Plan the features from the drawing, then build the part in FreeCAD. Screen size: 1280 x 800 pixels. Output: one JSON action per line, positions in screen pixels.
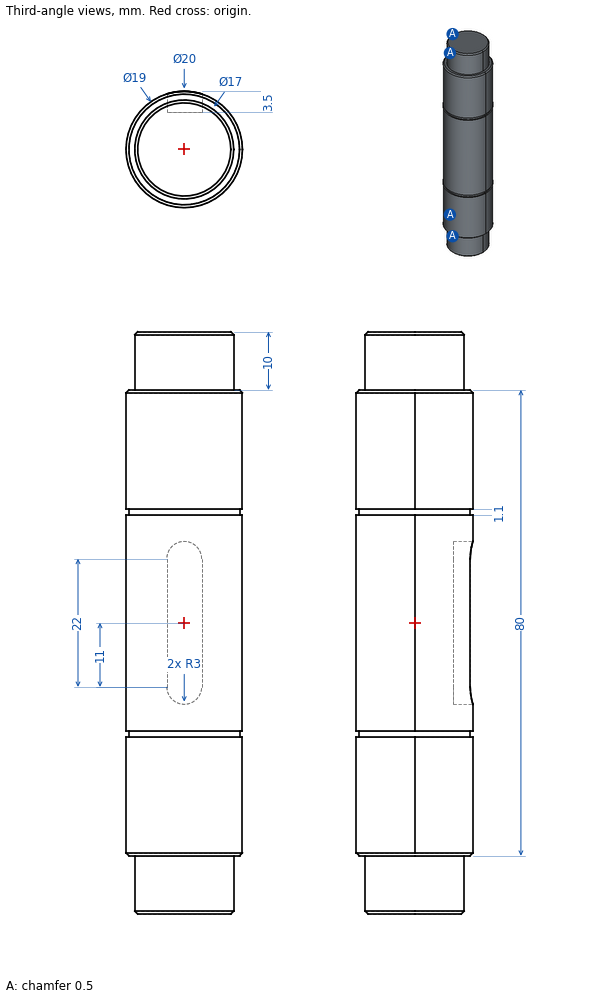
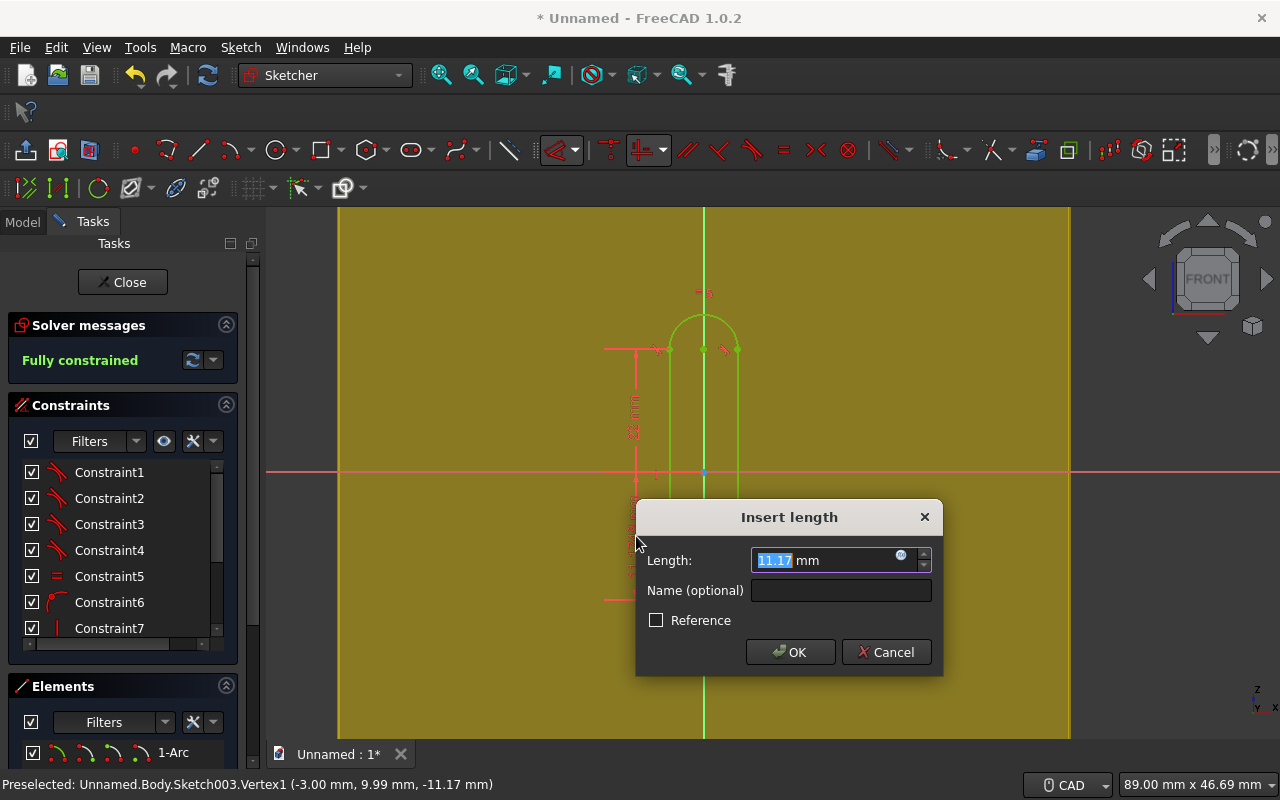
{"action": "type", "text": "11"}
{"action": "key", "text": "Return"}
{"action": "key", "text": "Escape"}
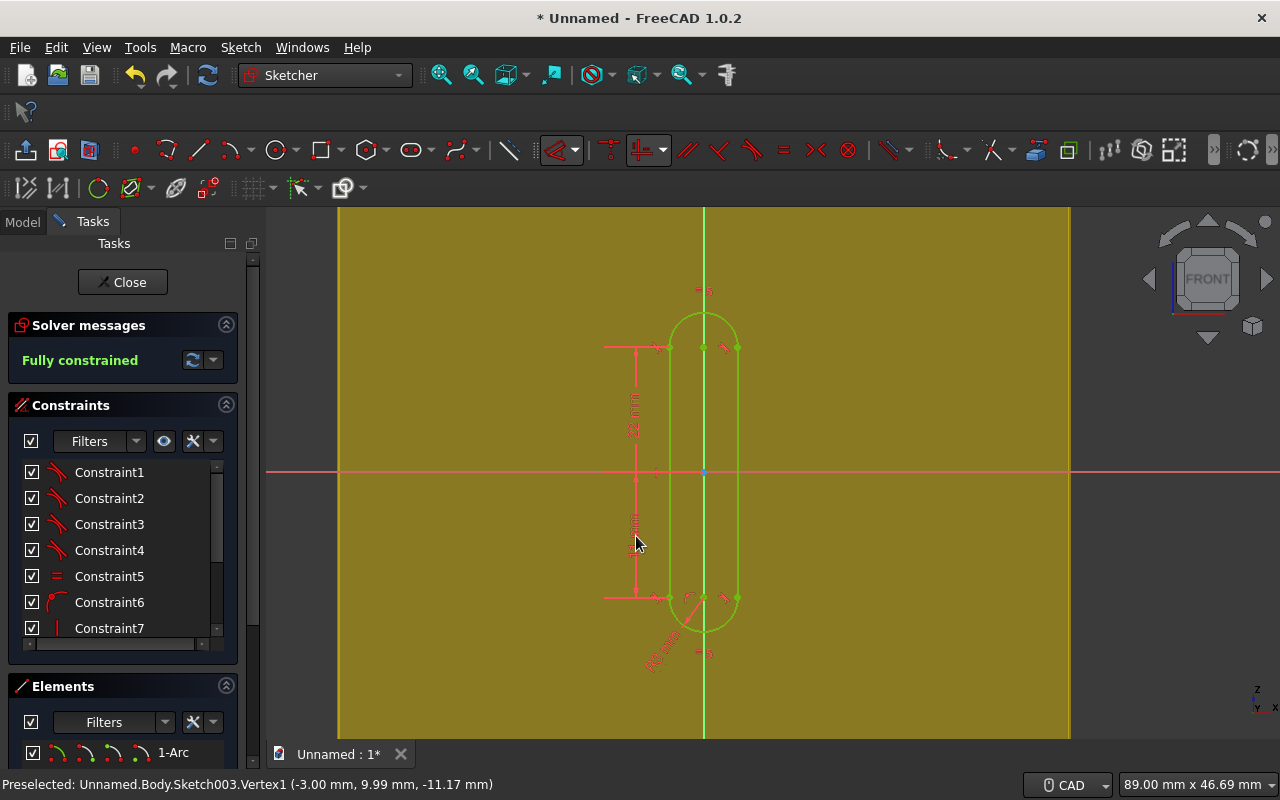
{"action": "left_click", "coordinate": [123, 282]}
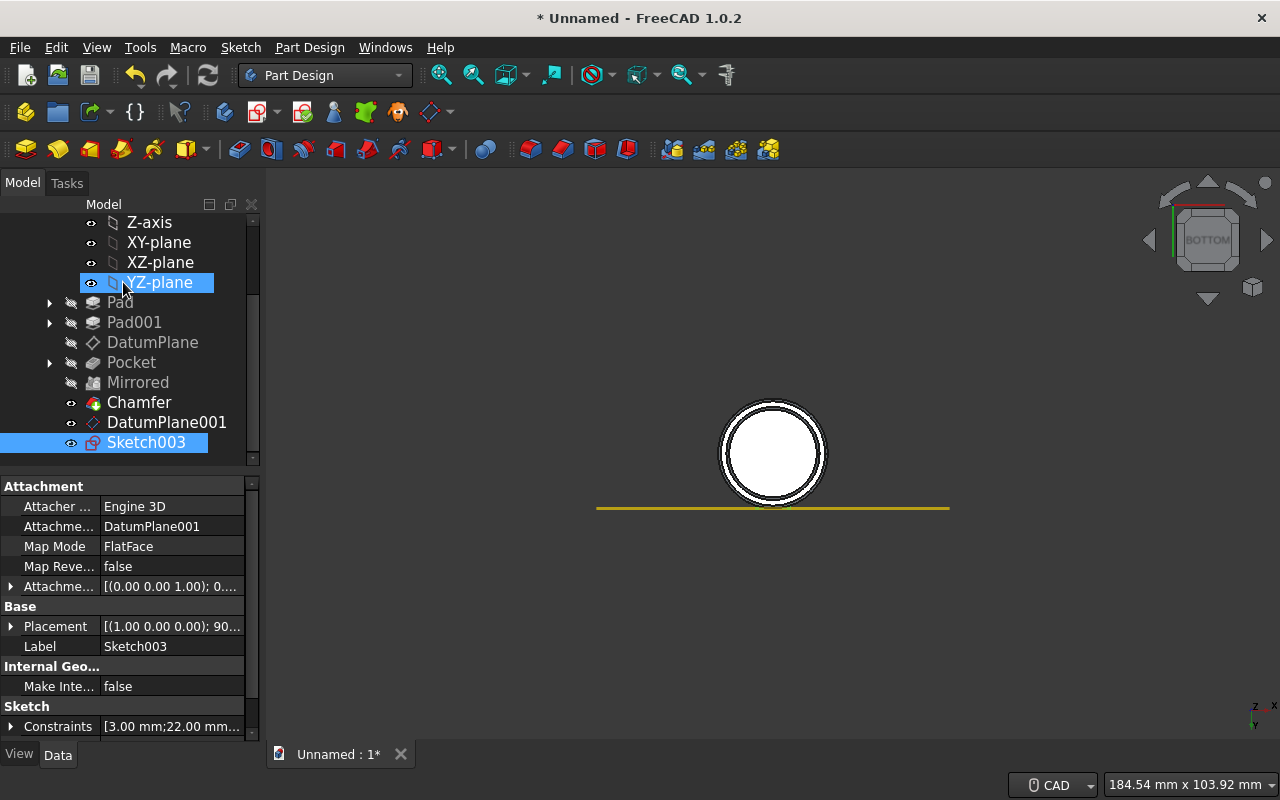
{"action": "left_click", "coordinate": [240, 150]}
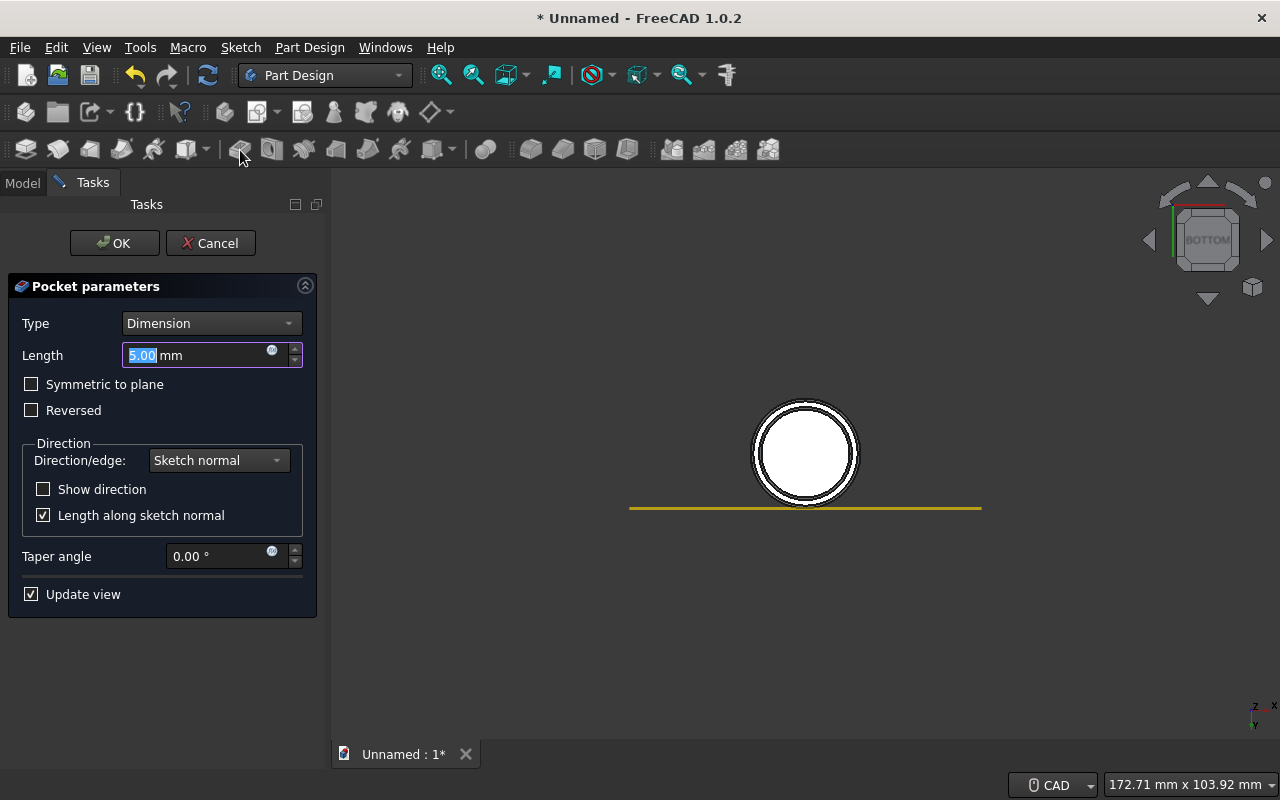
{"action": "type", "text": "3.5"}
{"action": "key", "text": "Tab"}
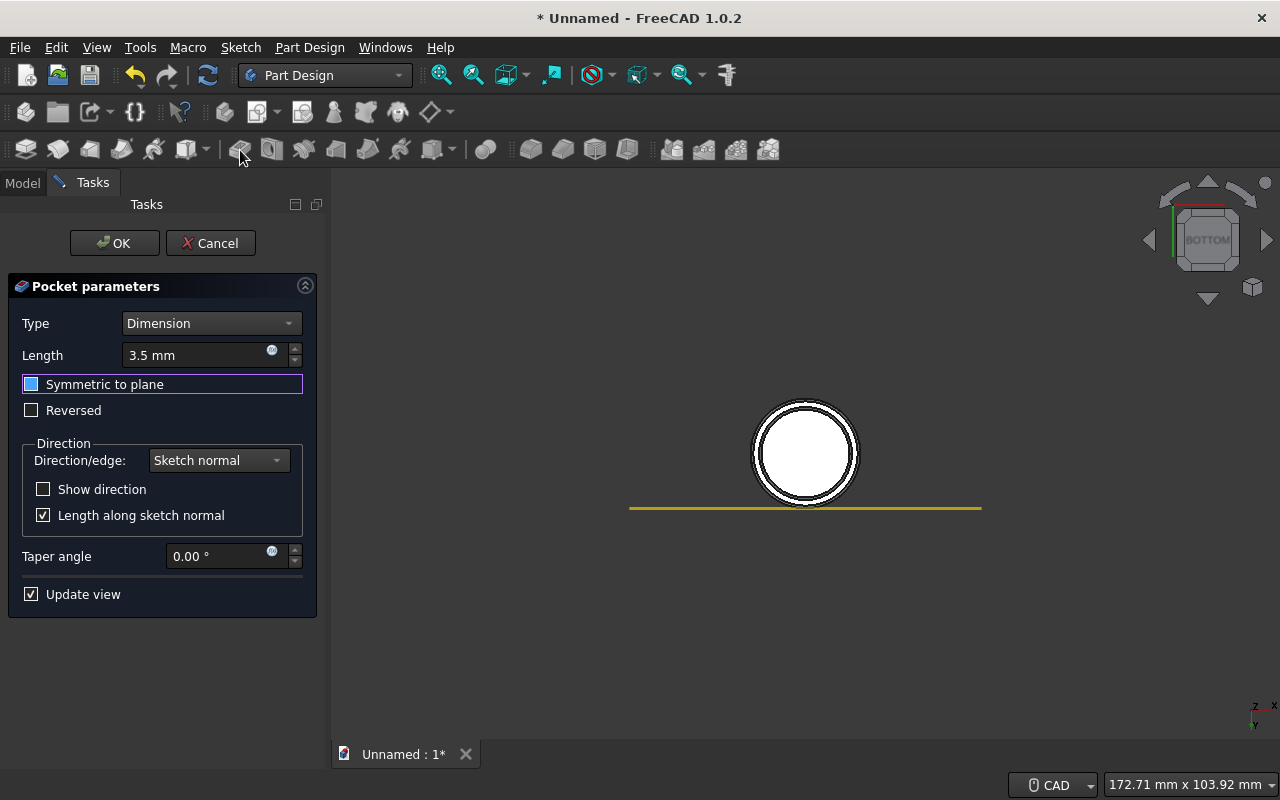
{"action": "left_click", "coordinate": [30, 410]}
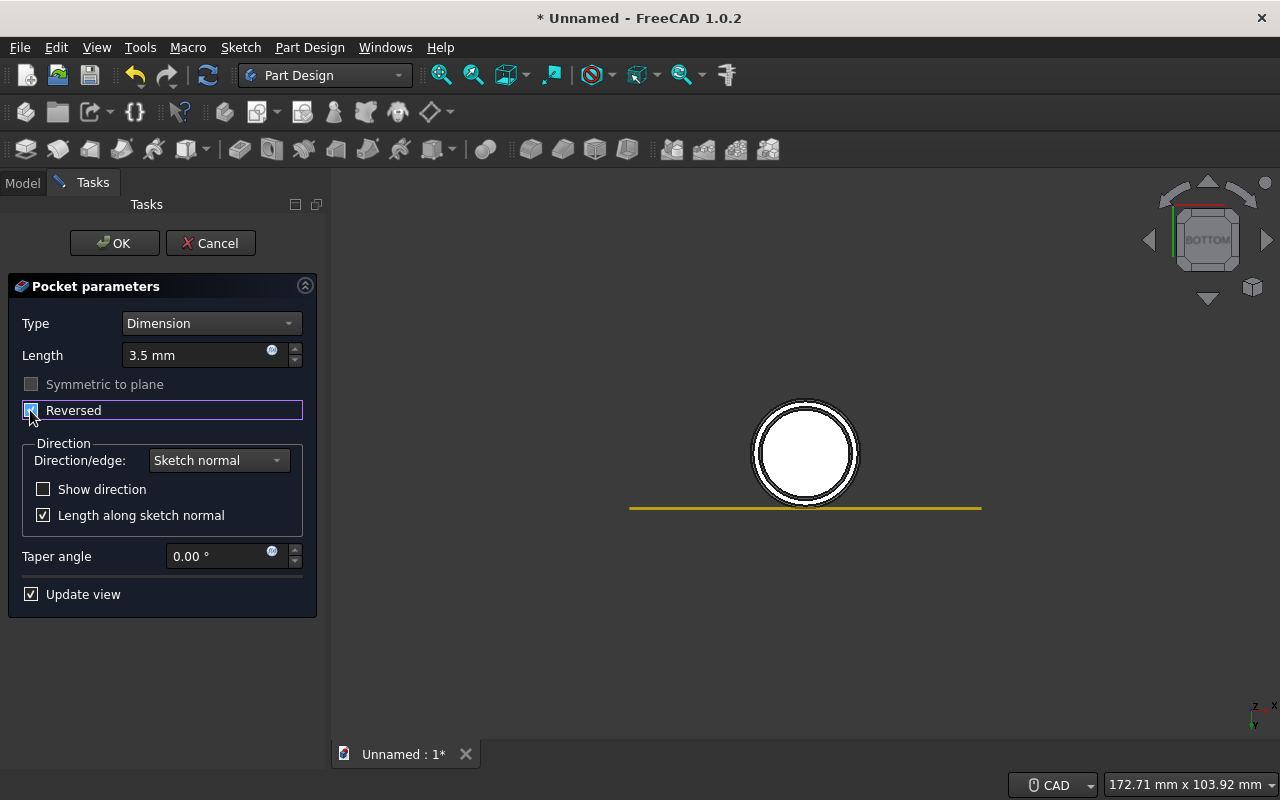
{"action": "left_click", "coordinate": [115, 243]}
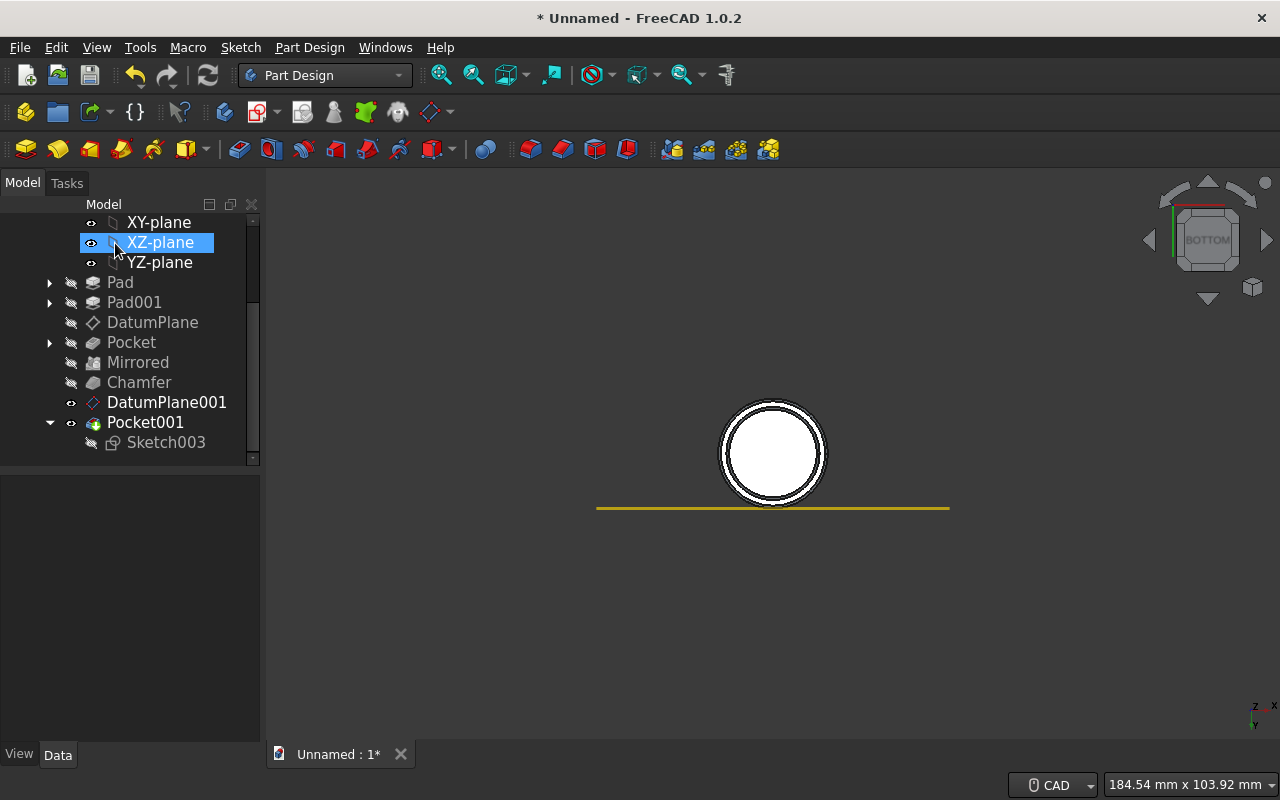
{"action": "left_click", "coordinate": [116, 403]}
{"action": "key", "text": "space"}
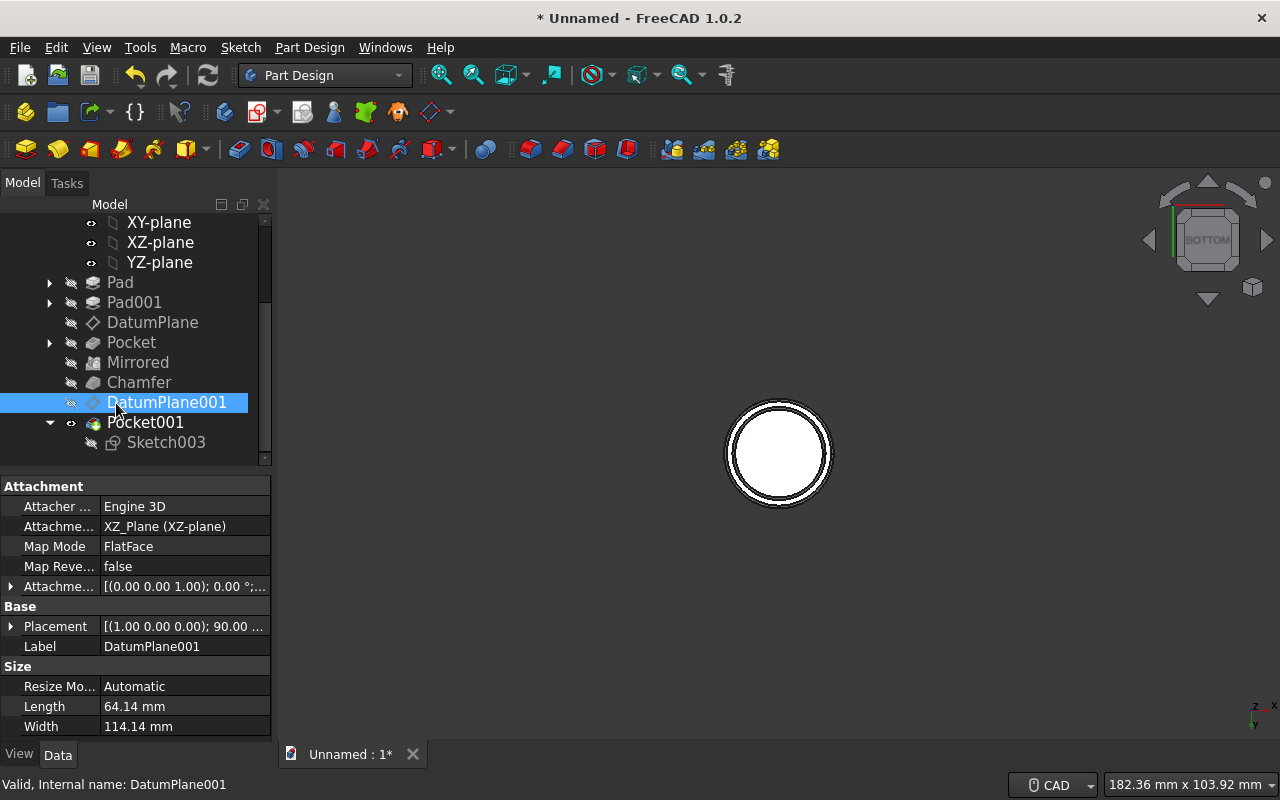
{"action": "key", "text": "0"}